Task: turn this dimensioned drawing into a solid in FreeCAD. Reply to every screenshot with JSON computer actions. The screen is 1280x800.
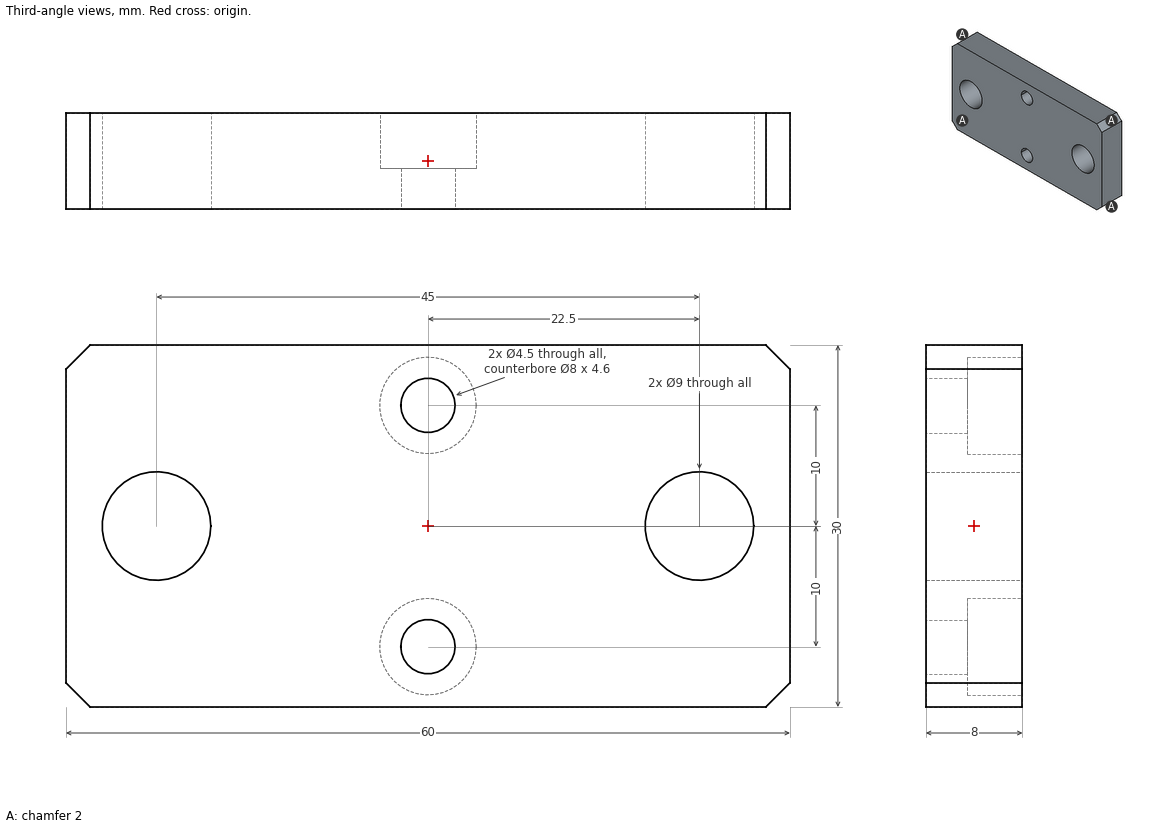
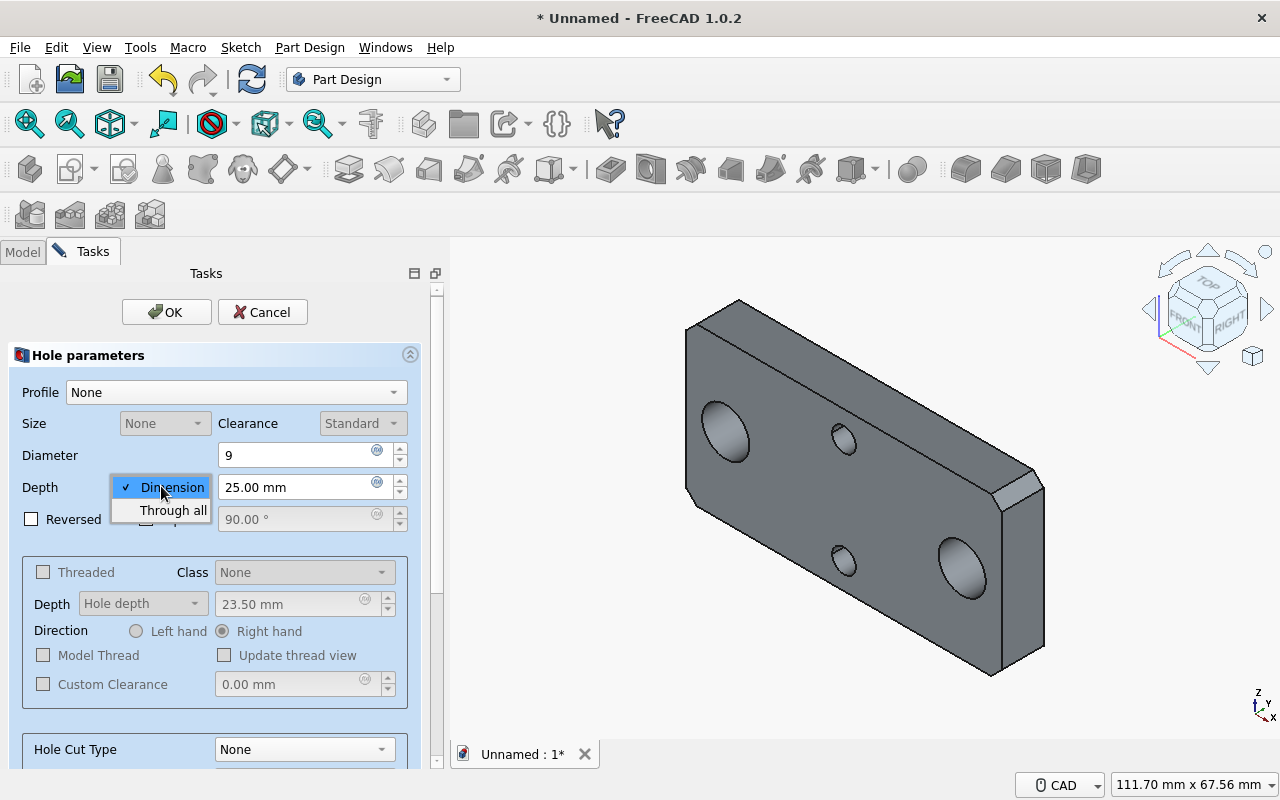
{"action": "left_click", "coordinate": [160, 510]}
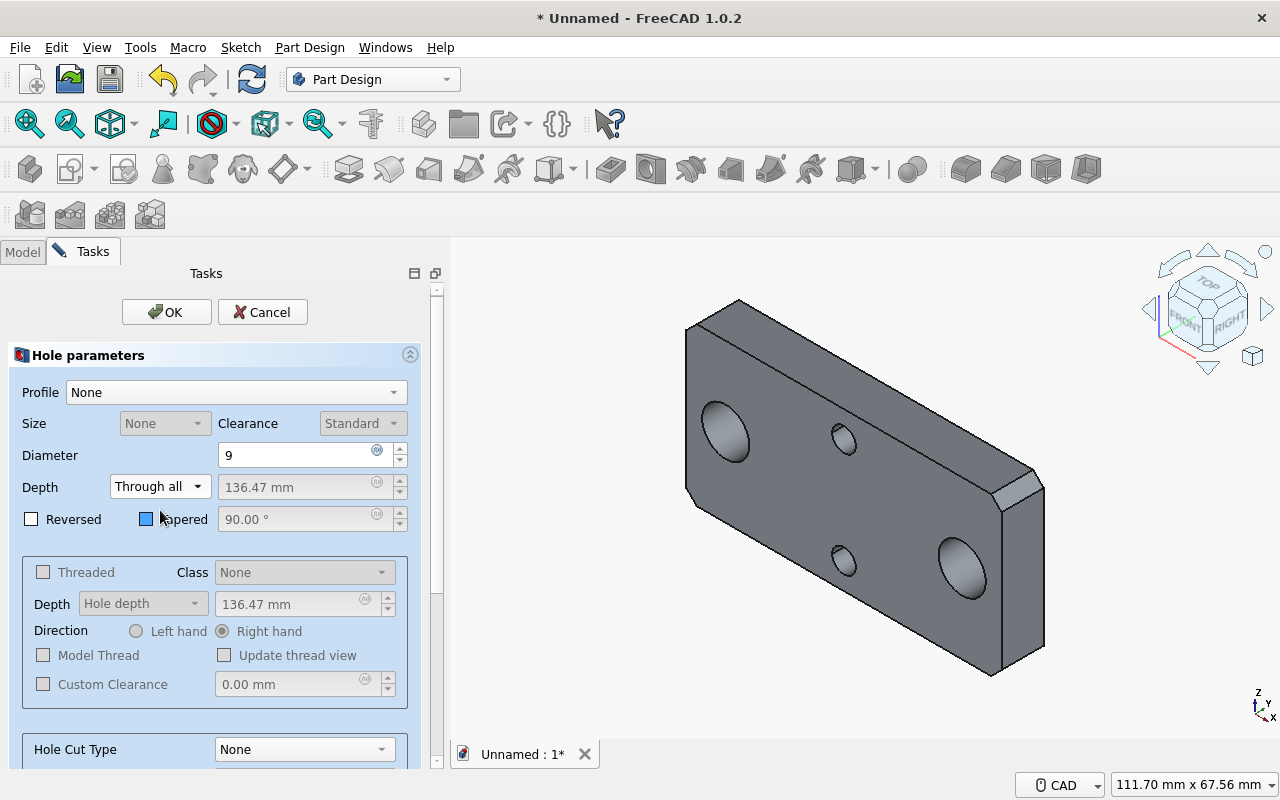
{"action": "left_click", "coordinate": [167, 312]}